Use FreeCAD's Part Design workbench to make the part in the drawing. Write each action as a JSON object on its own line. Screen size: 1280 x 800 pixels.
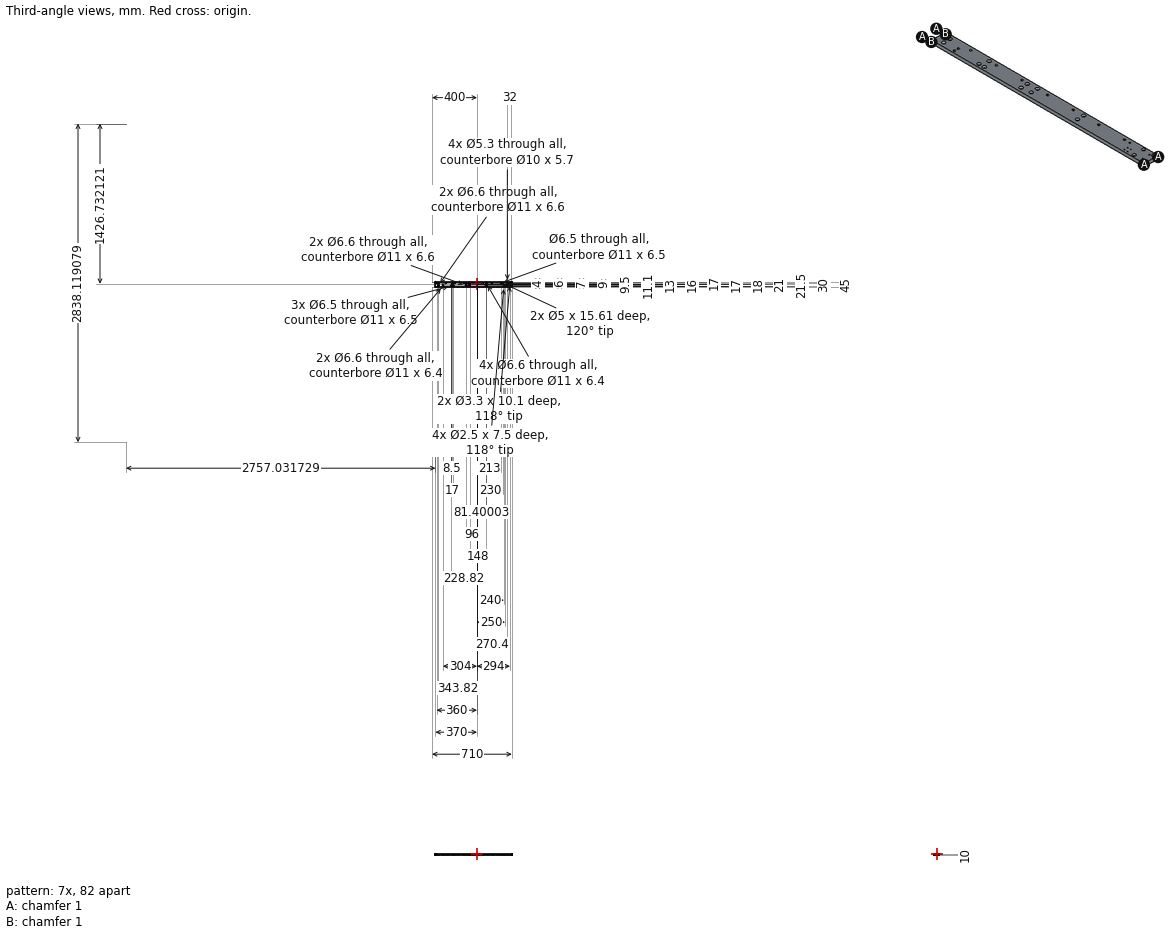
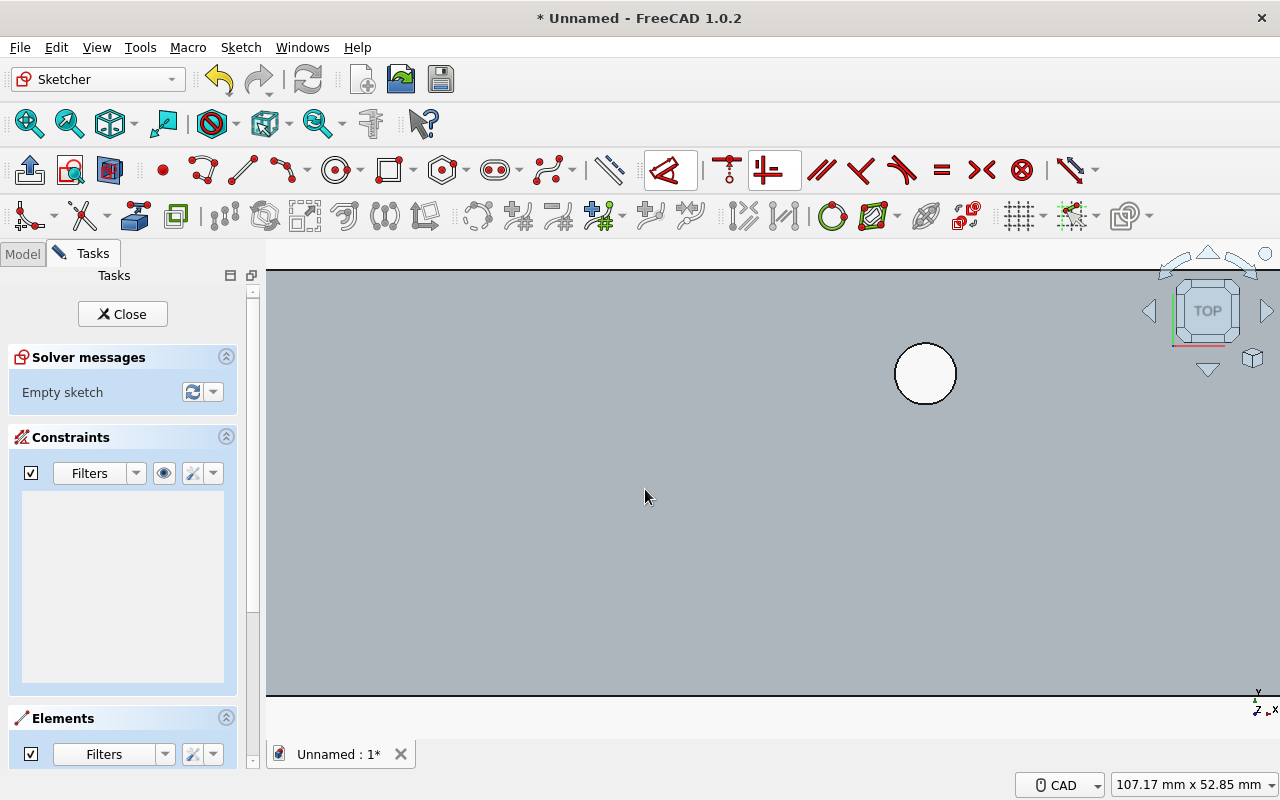
{"action": "left_click", "coordinate": [336, 170]}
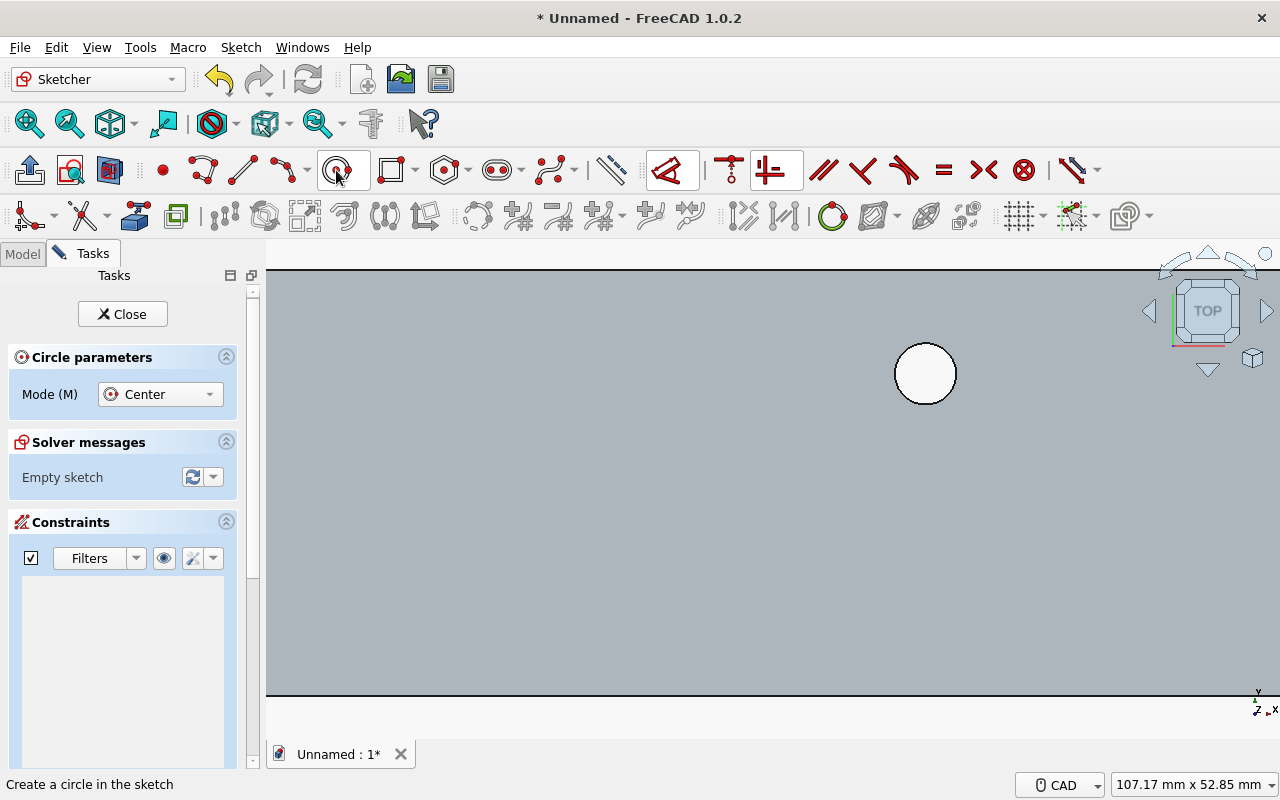
{"action": "left_click", "coordinate": [624, 601]}
{"action": "left_click", "coordinate": [646, 579]}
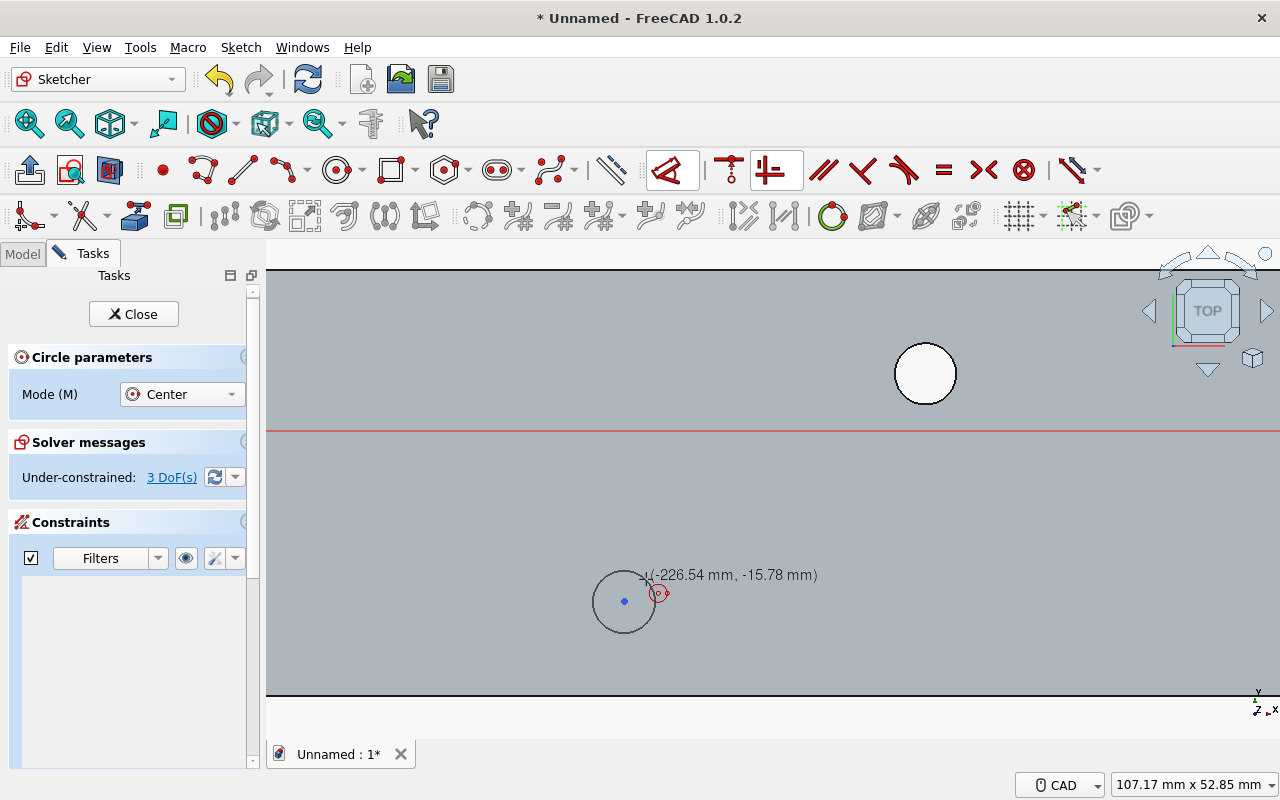
{"action": "left_click", "coordinate": [785, 601]}
{"action": "left_click", "coordinate": [807, 579]}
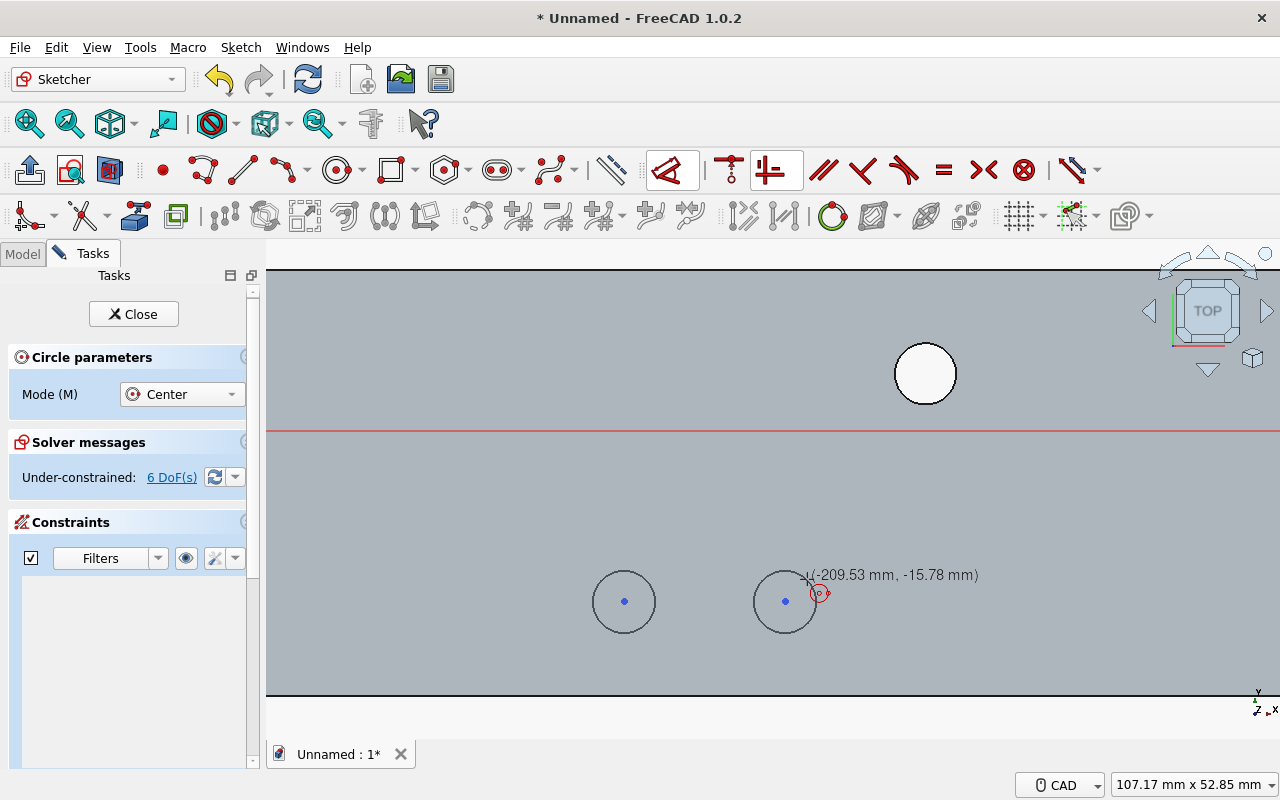
{"action": "left_click", "coordinate": [705, 374]}
{"action": "left_click", "coordinate": [727, 352]}
{"action": "key", "text": "Escape"}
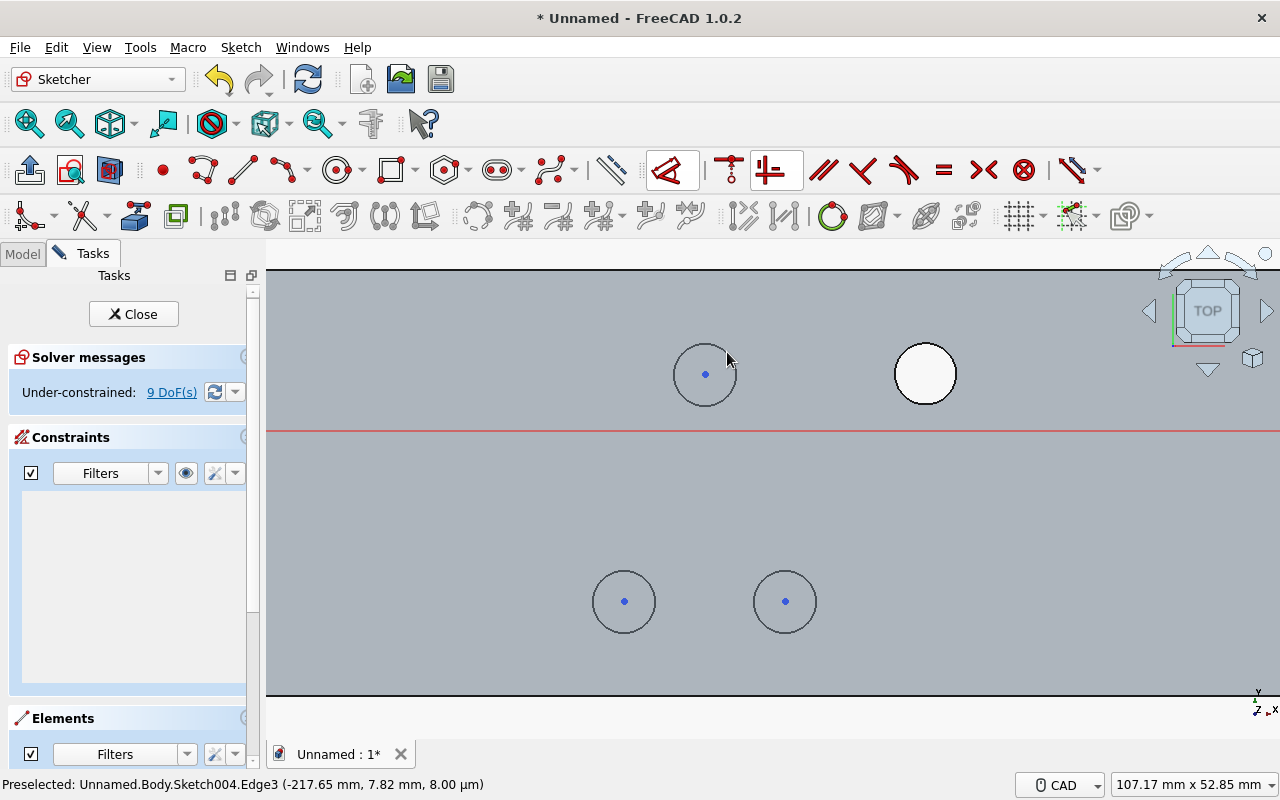
{"action": "left_click", "coordinate": [646, 580]}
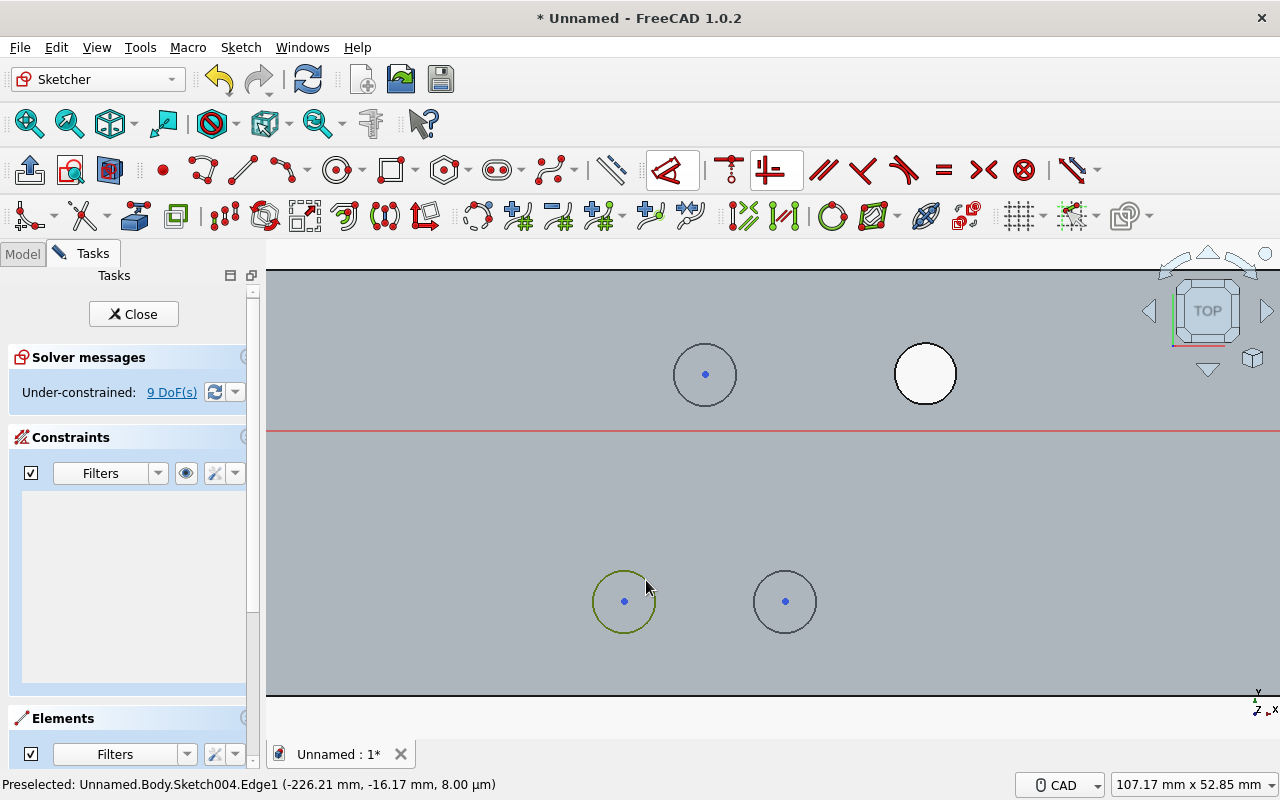
{"action": "left_click", "coordinate": [807, 580]}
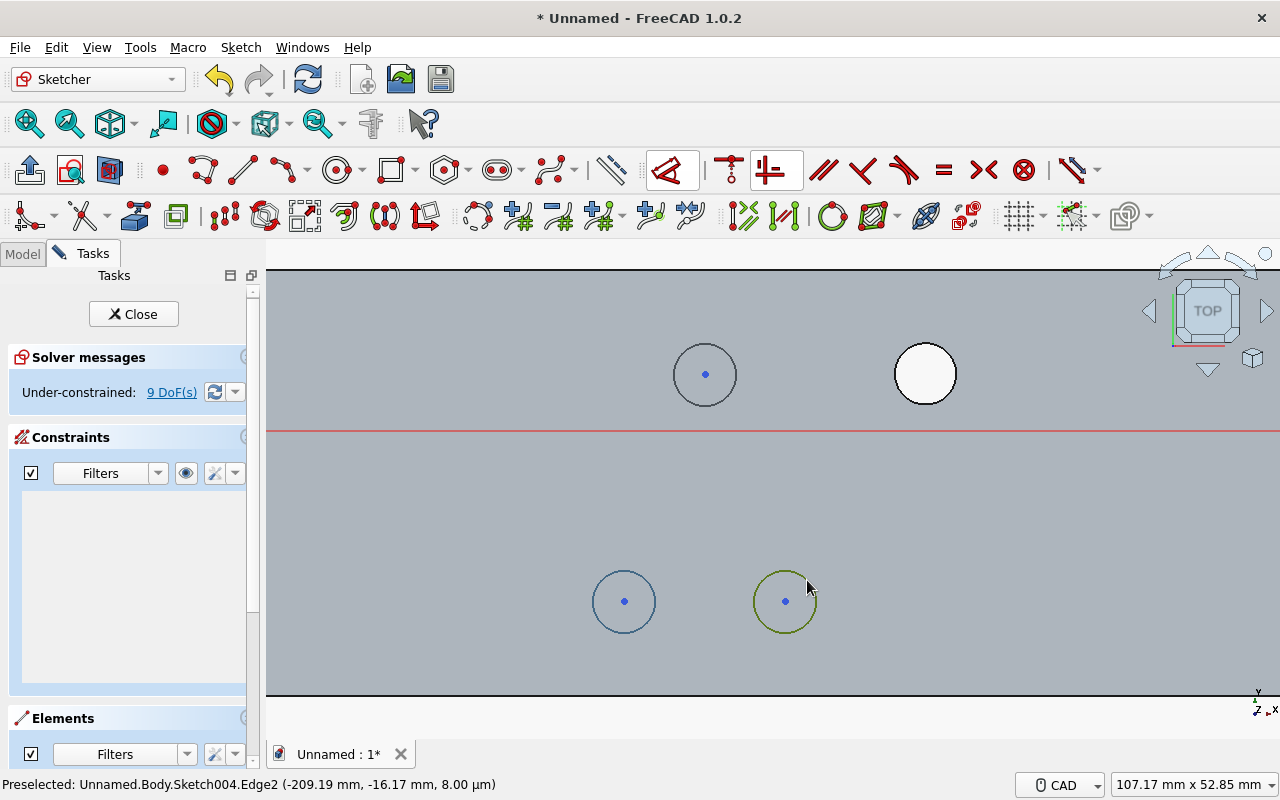
{"action": "left_click", "coordinate": [727, 353]}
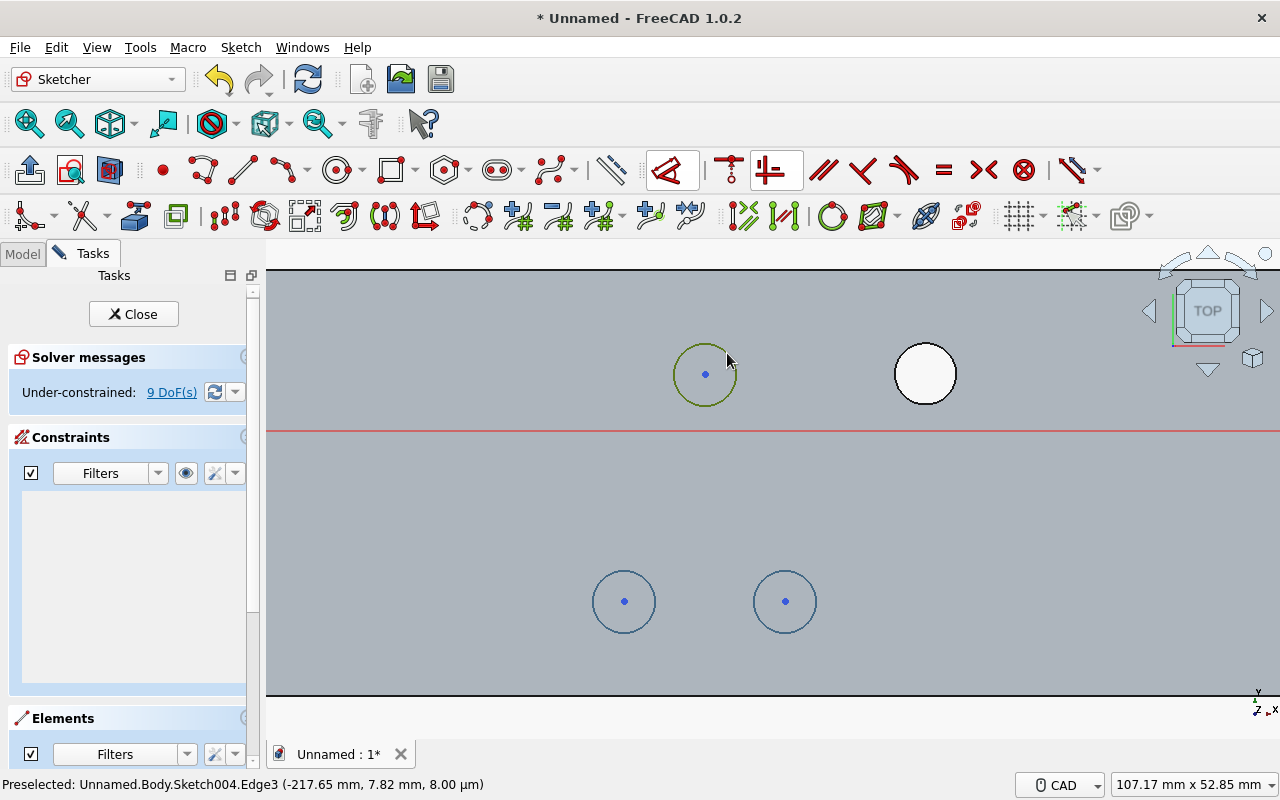
{"action": "left_click", "coordinate": [944, 170]}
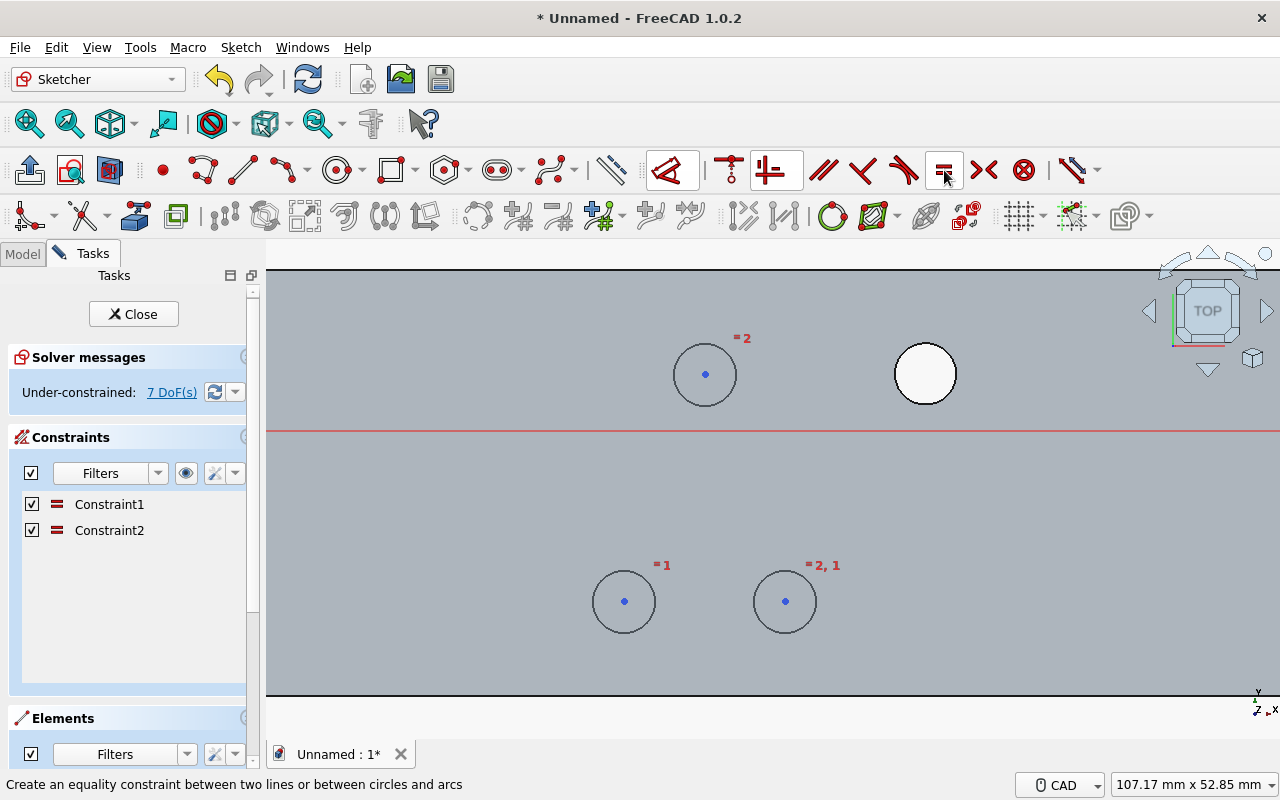
{"action": "left_click", "coordinate": [624, 602]}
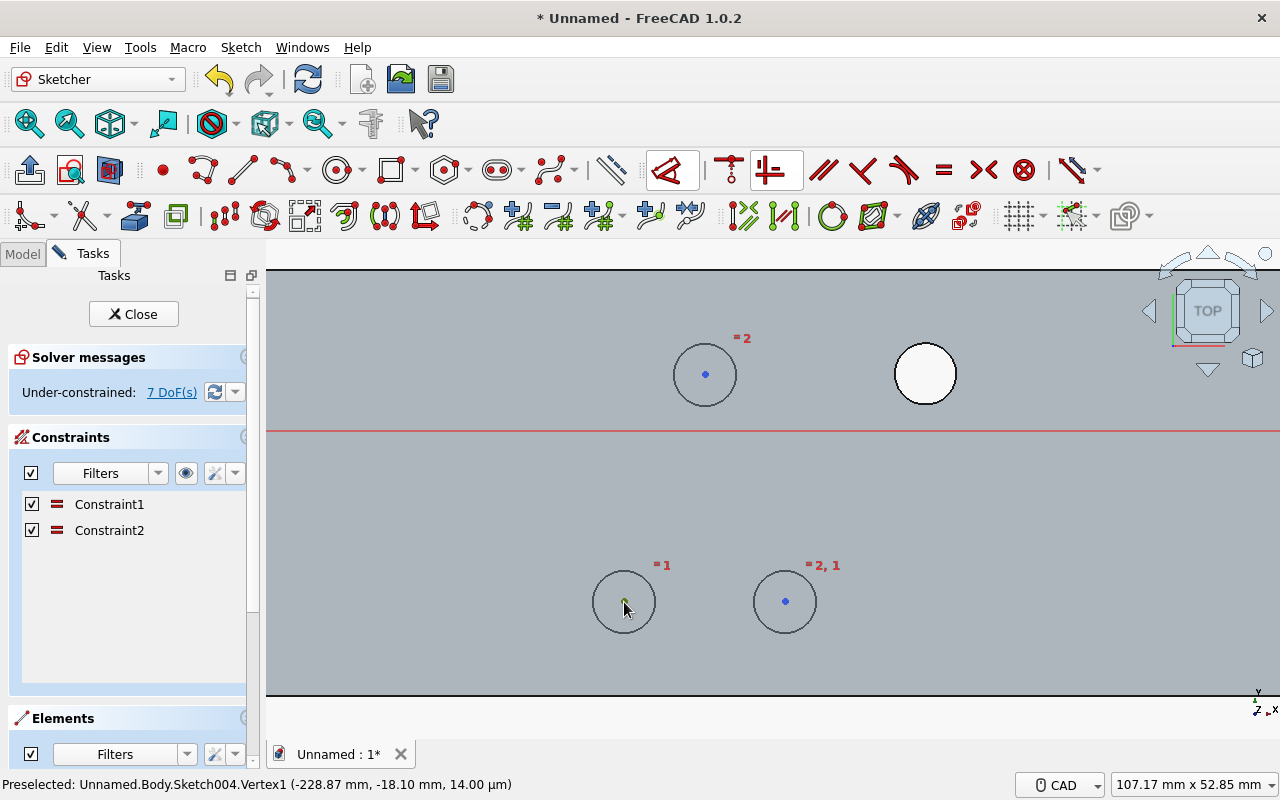
{"action": "left_click", "coordinate": [785, 602]}